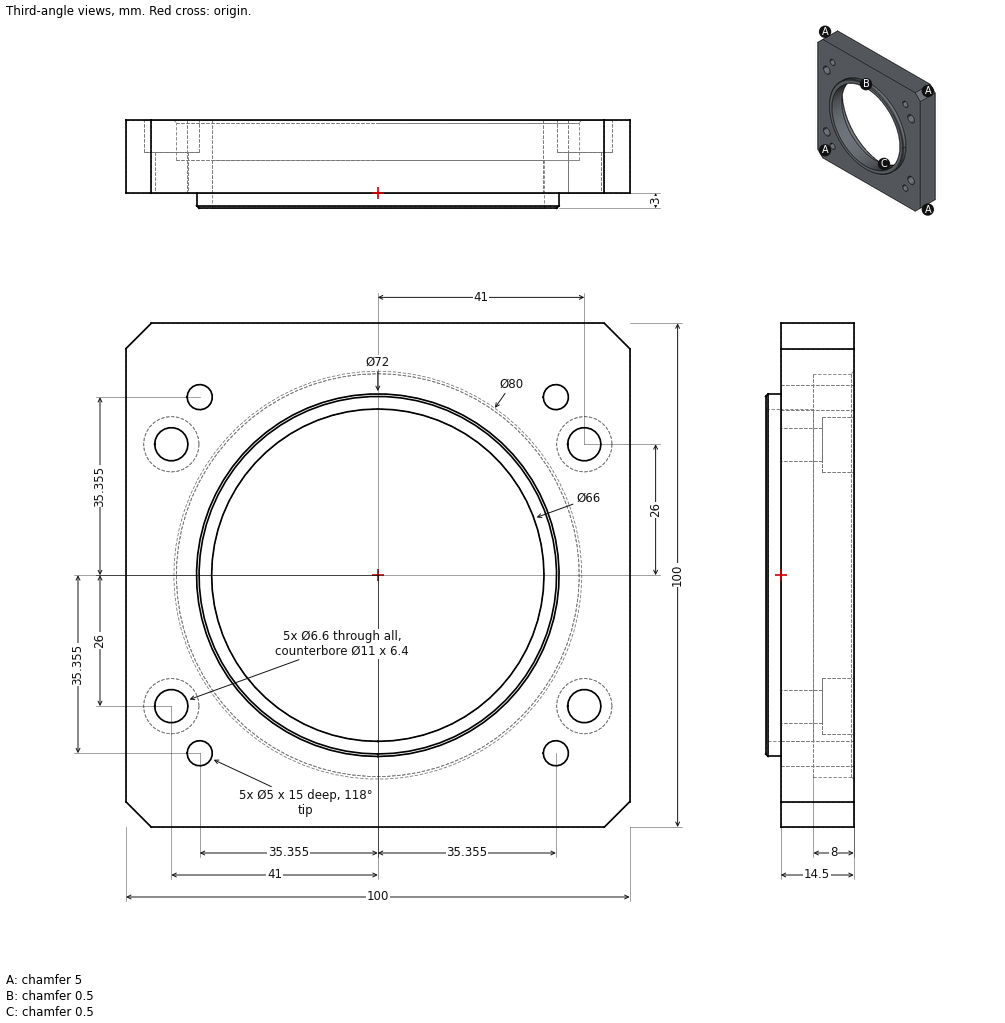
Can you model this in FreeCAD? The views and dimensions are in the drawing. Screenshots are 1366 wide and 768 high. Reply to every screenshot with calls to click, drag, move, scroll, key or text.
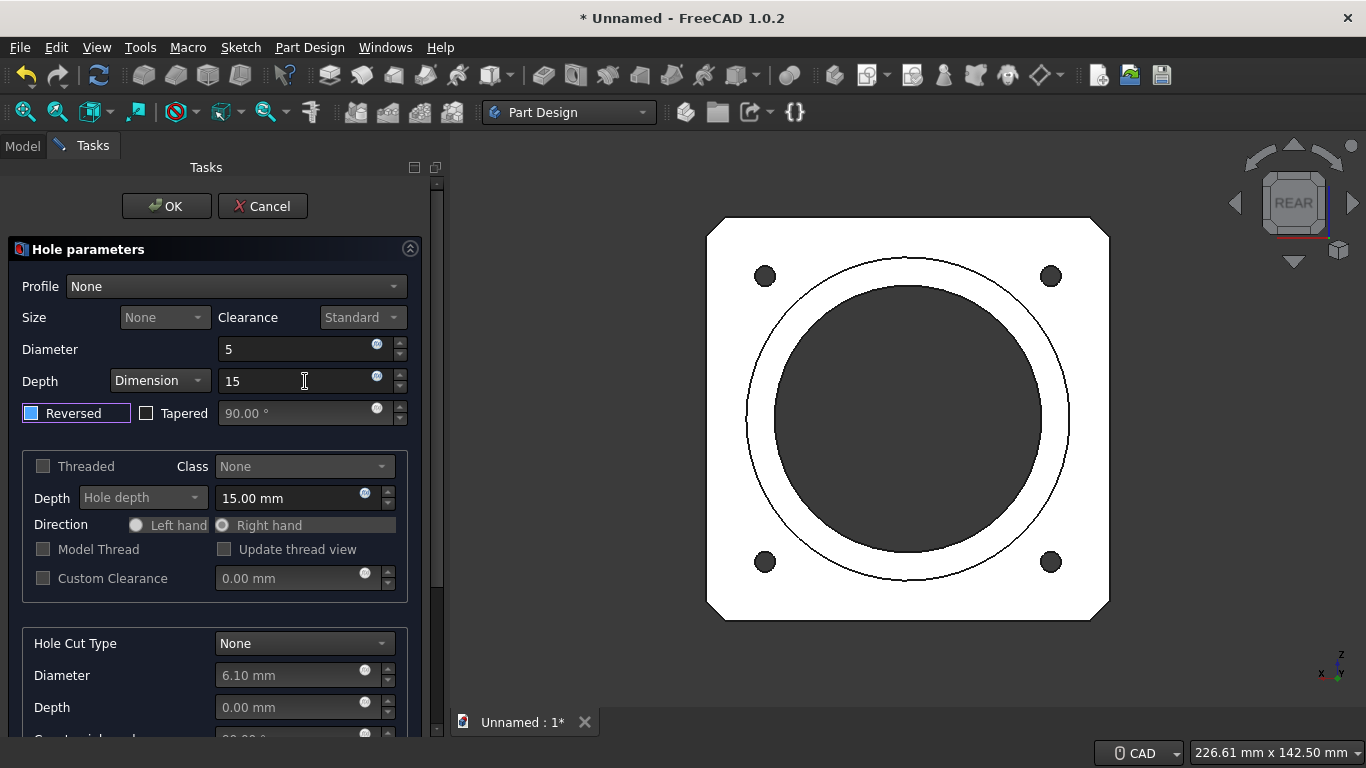
click(167, 206)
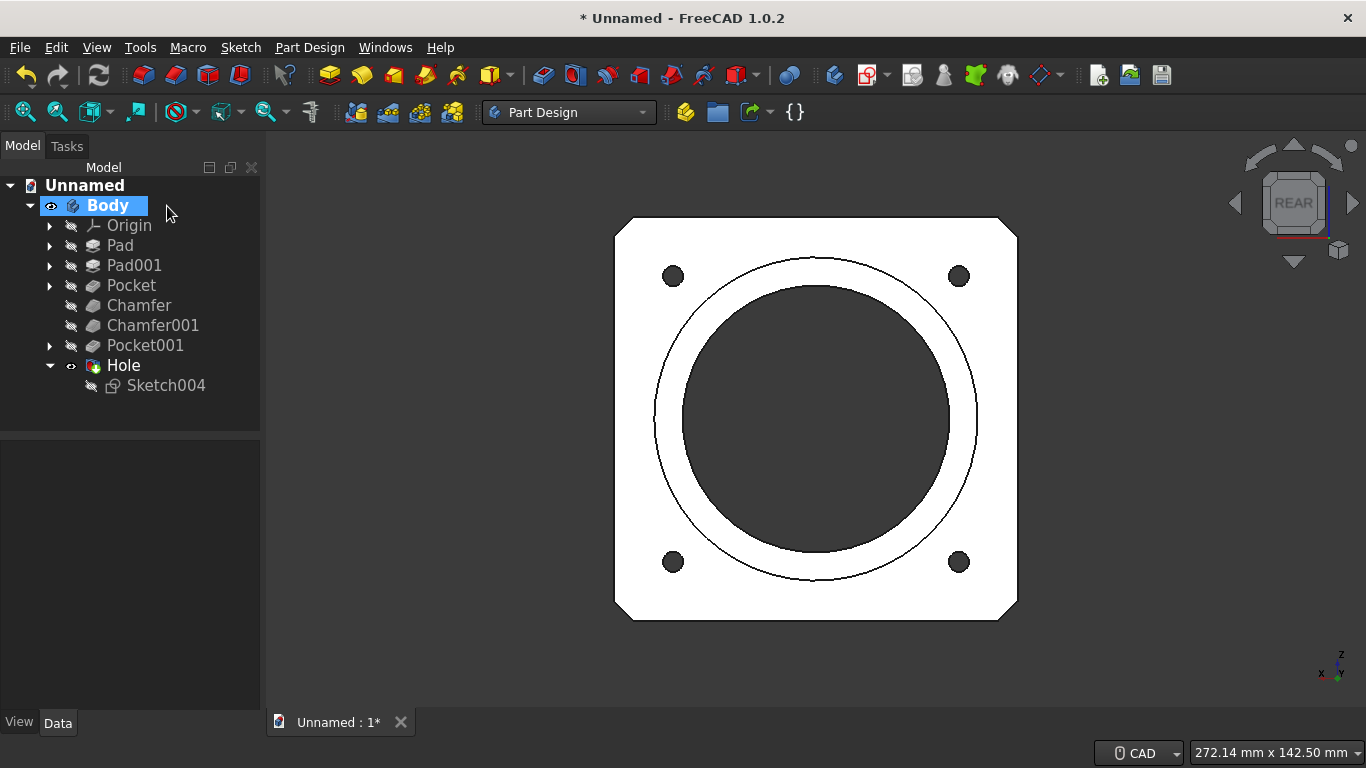
click(701, 245)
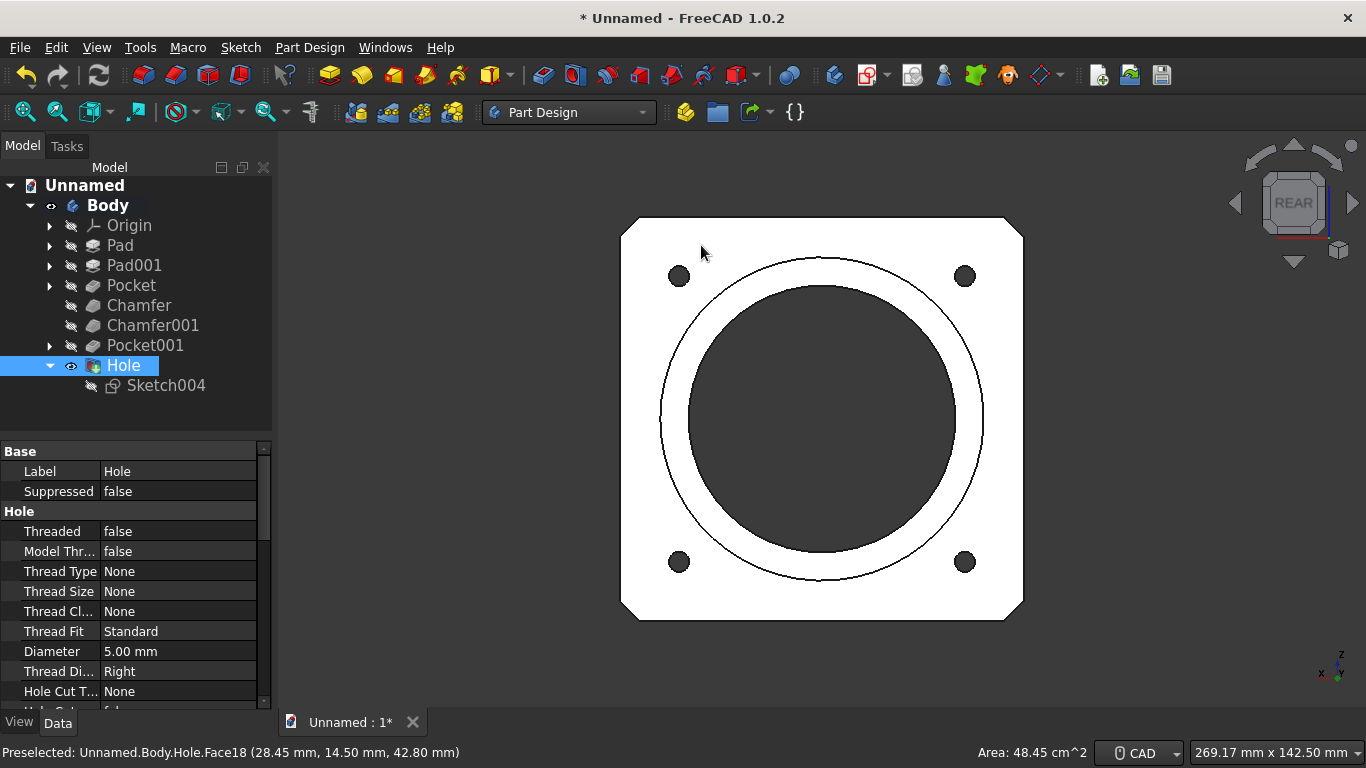
click(868, 76)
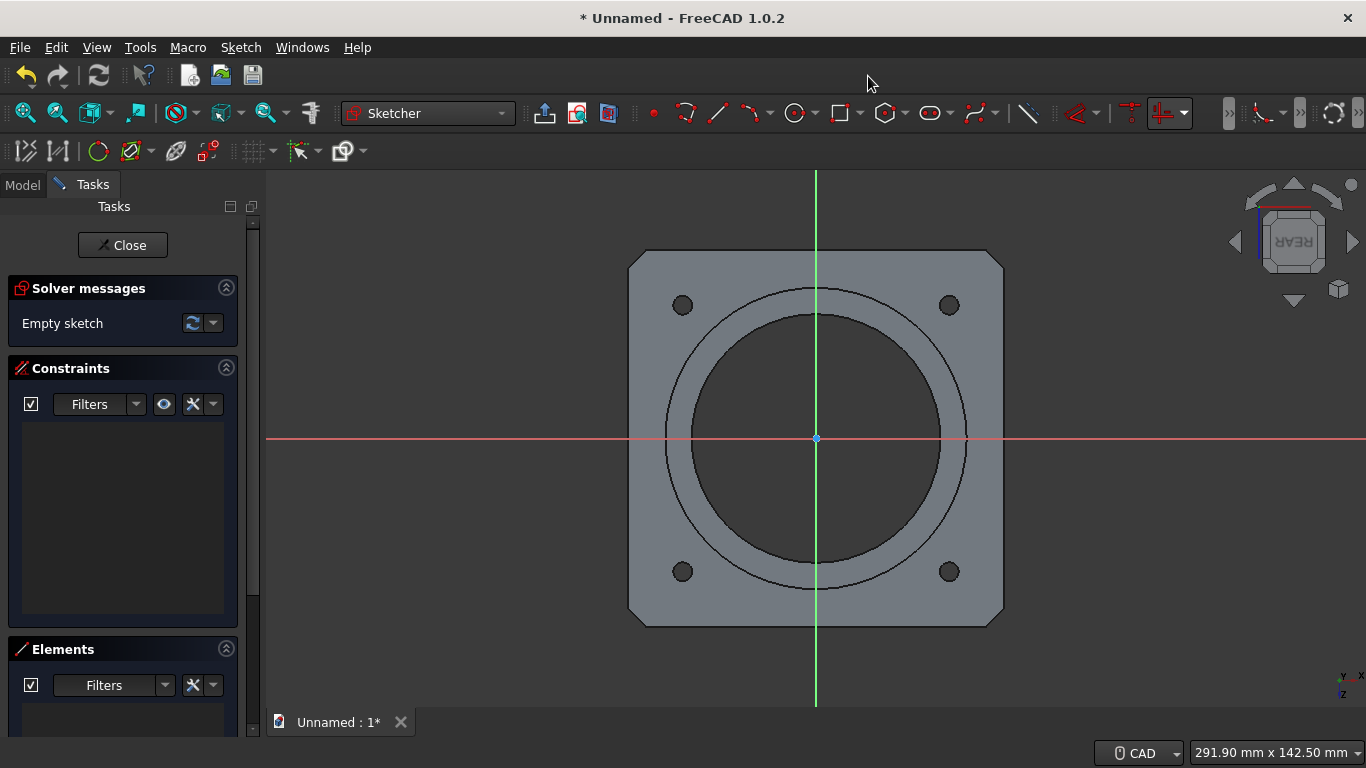
scroll(955, 438, up, 2)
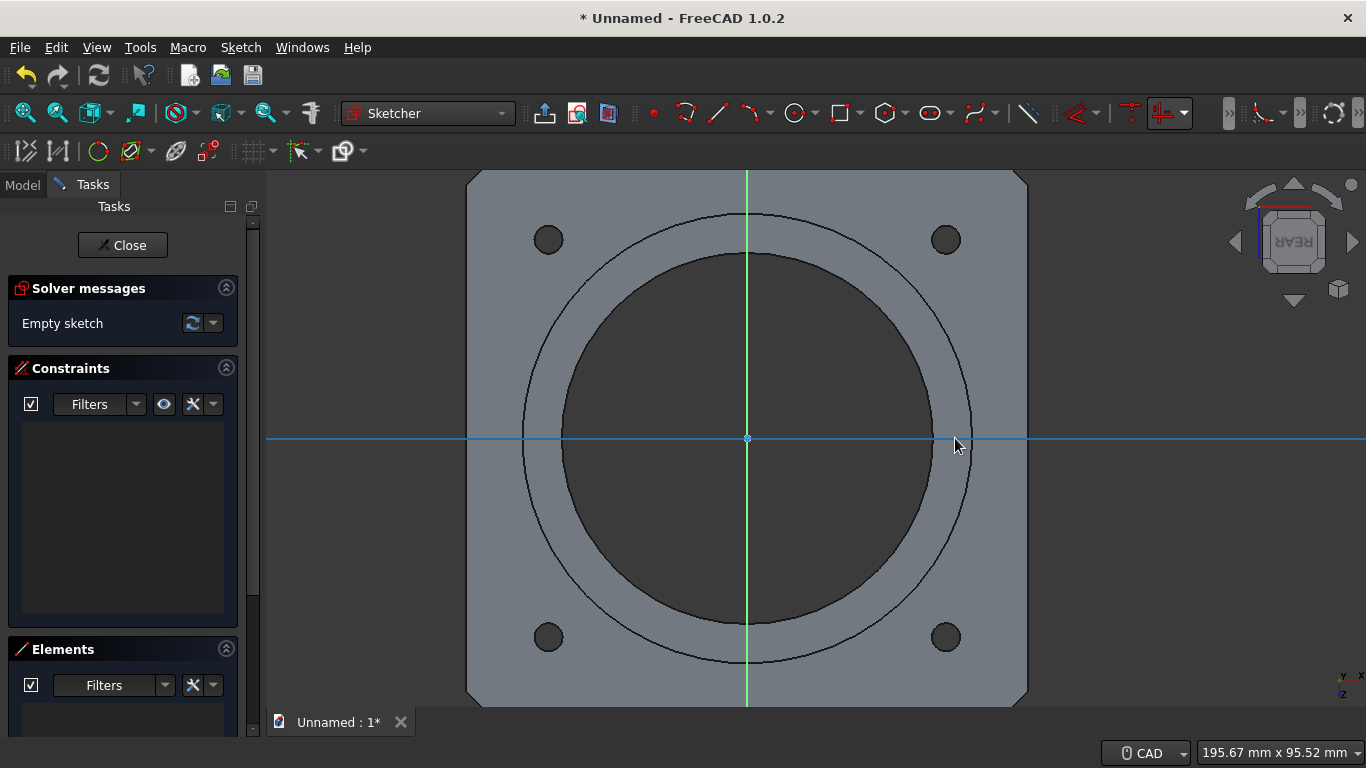
key(g)
key(c)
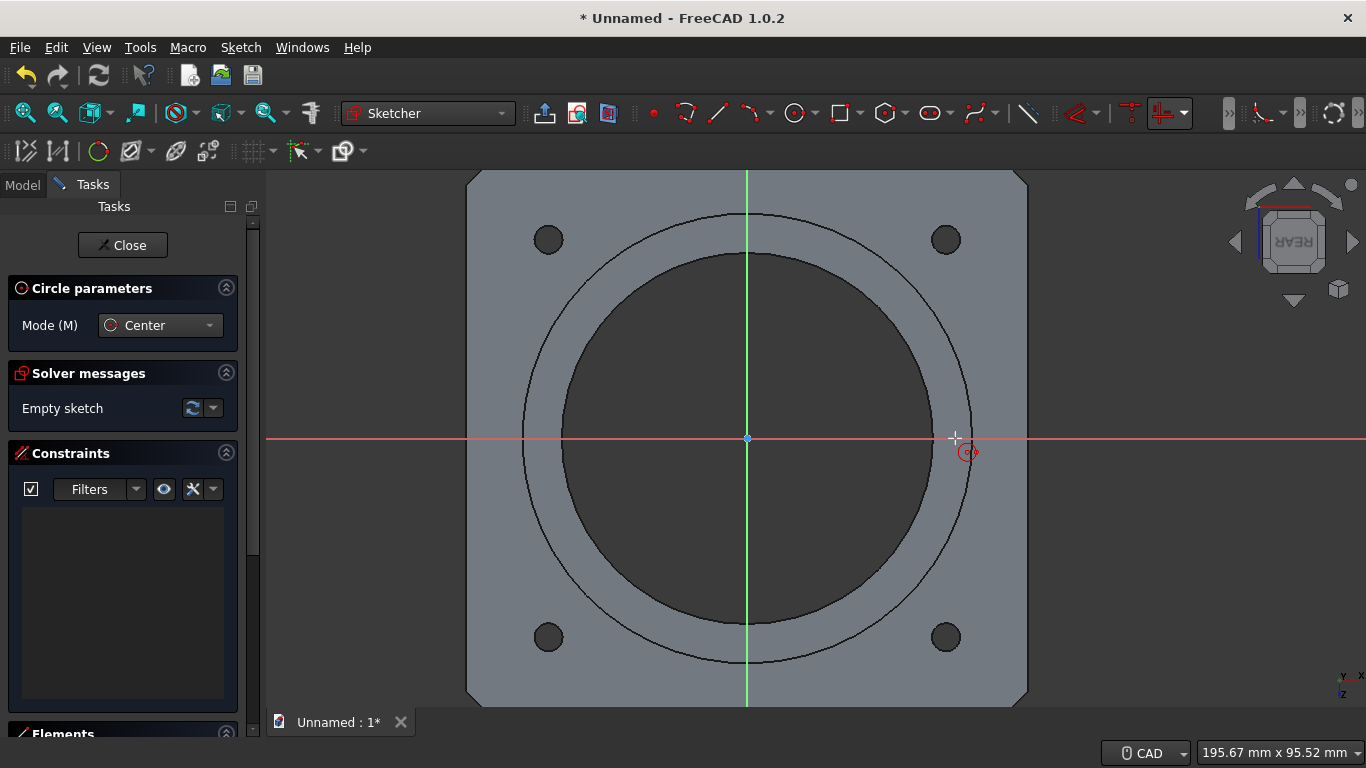
scroll(517, 292, up, 2)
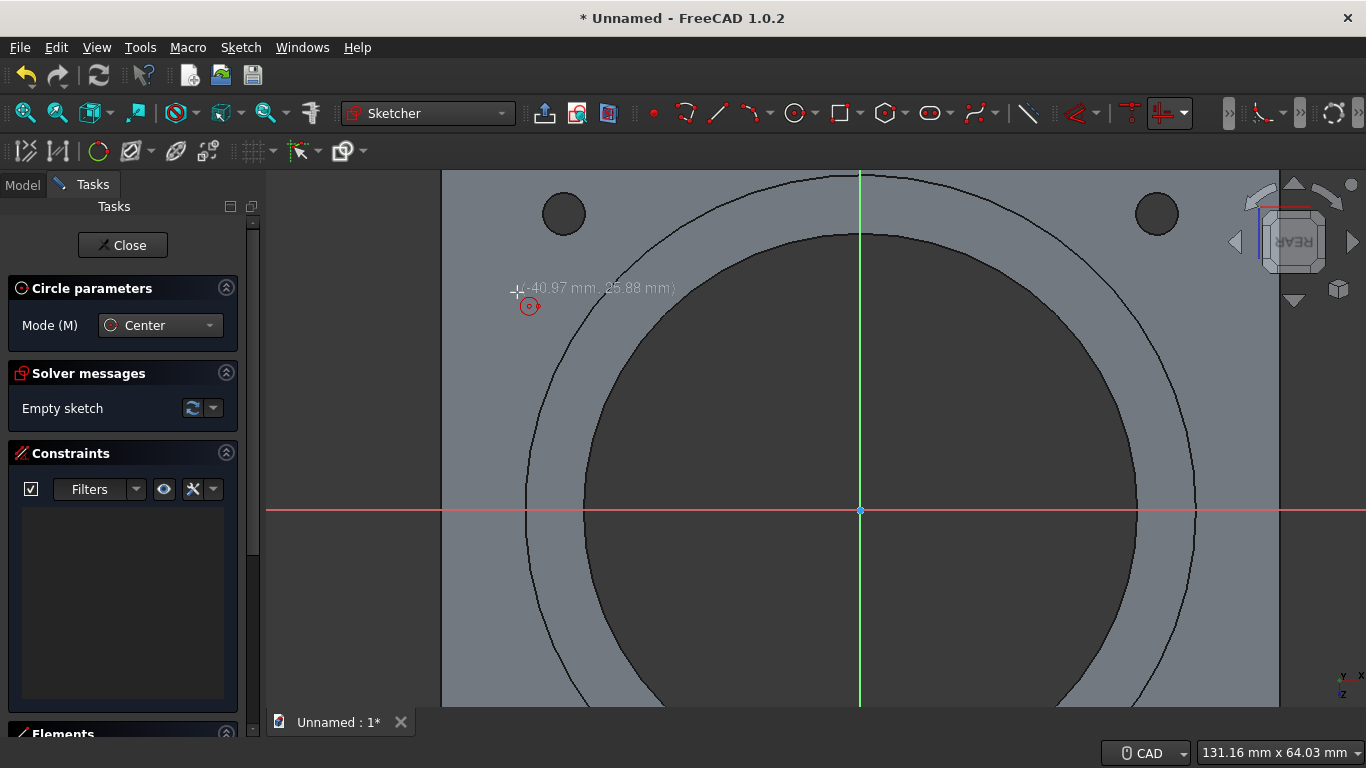
click(517, 292)
click(536, 273)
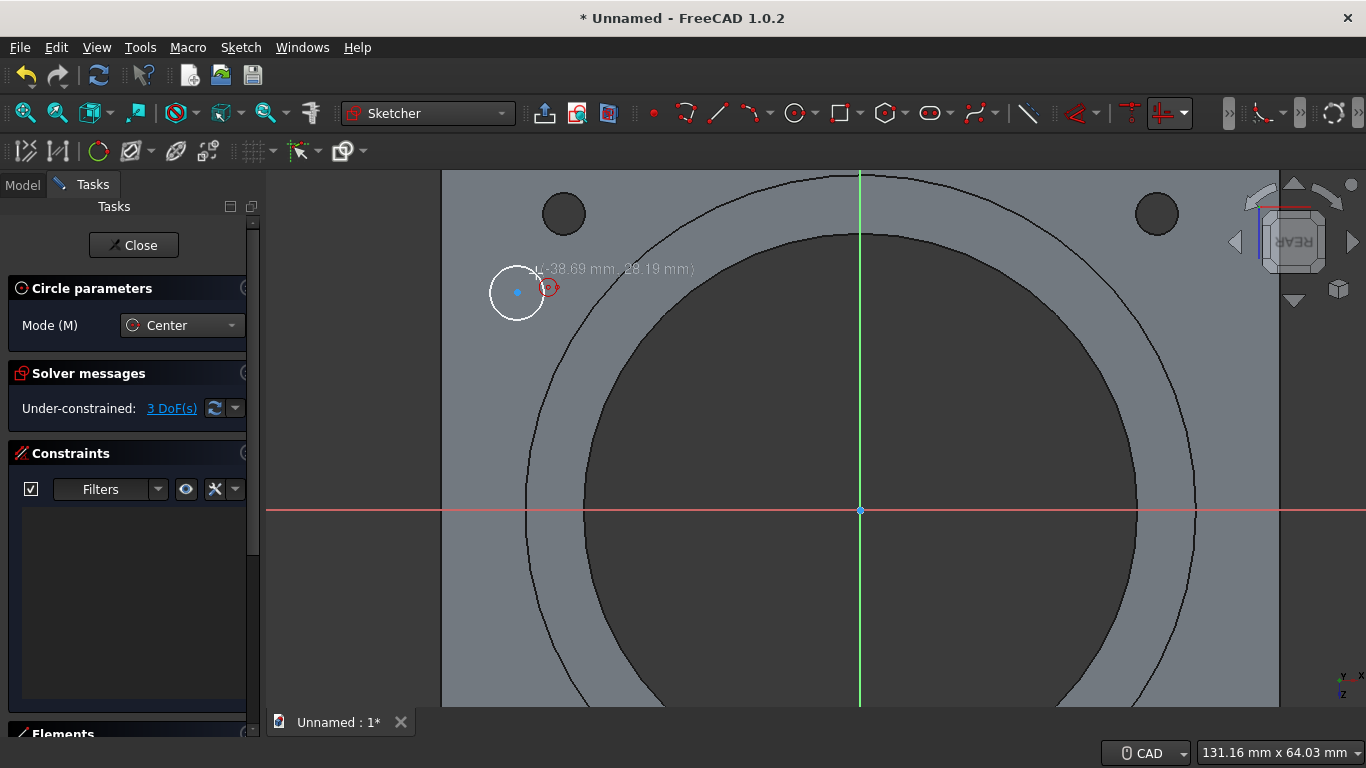
click(860, 510)
click(880, 491)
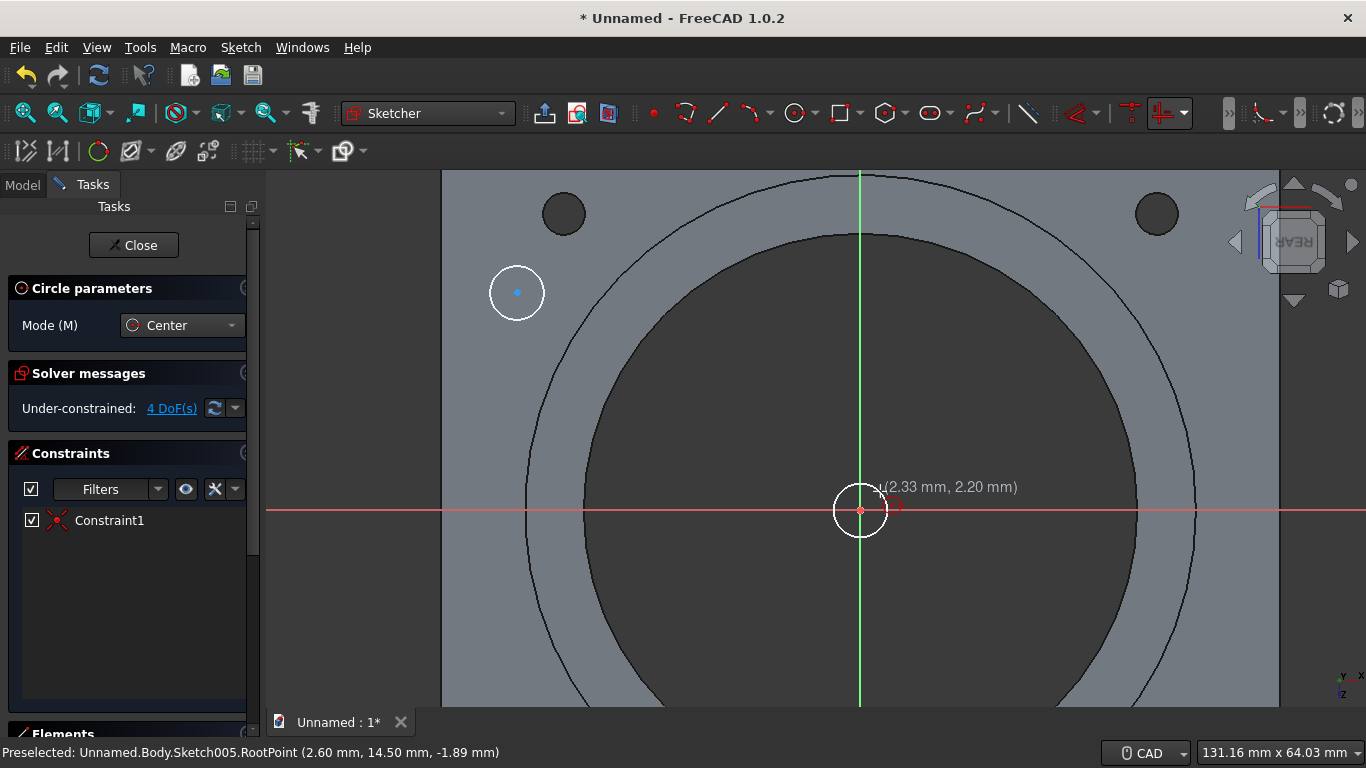
scroll(518, 292, down, 2)